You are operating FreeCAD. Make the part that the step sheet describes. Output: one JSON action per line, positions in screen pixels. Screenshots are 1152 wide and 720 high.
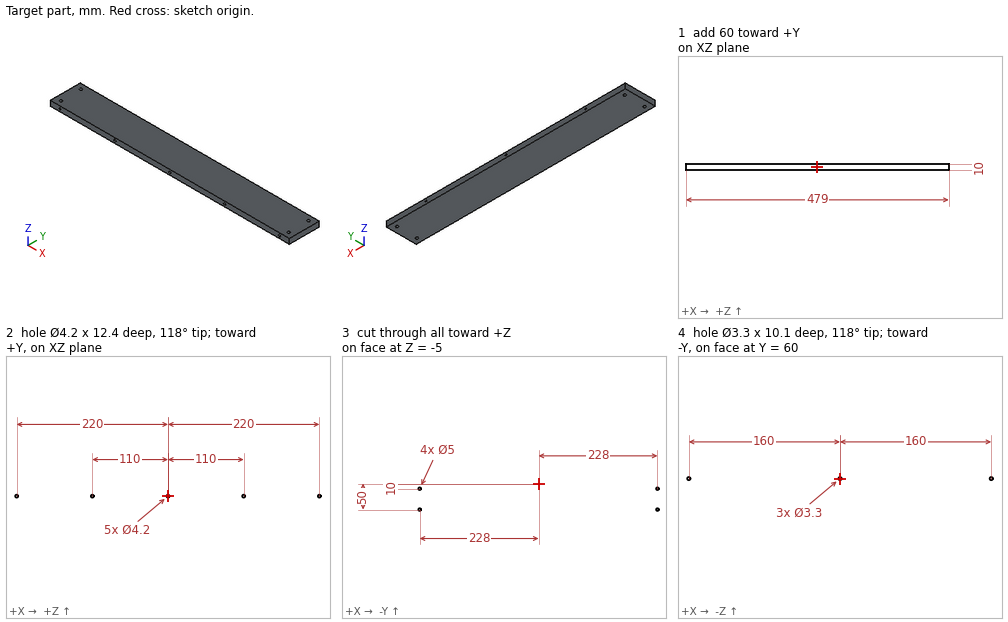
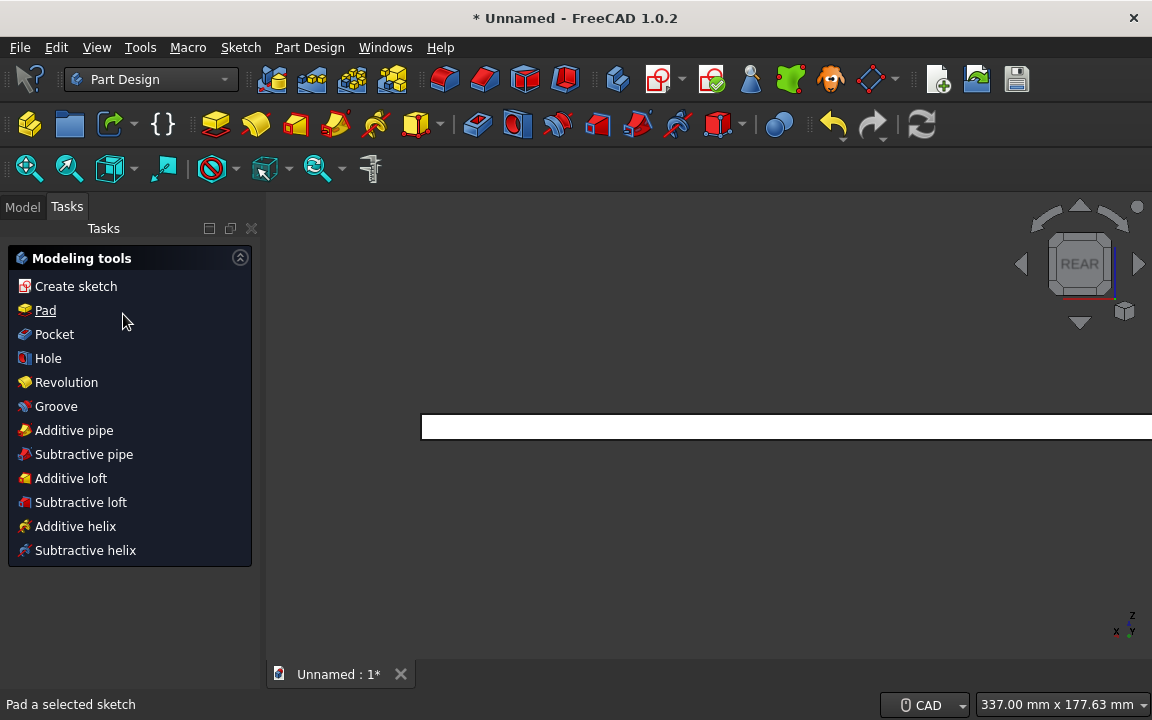
{"action": "left_click", "coordinate": [518, 124]}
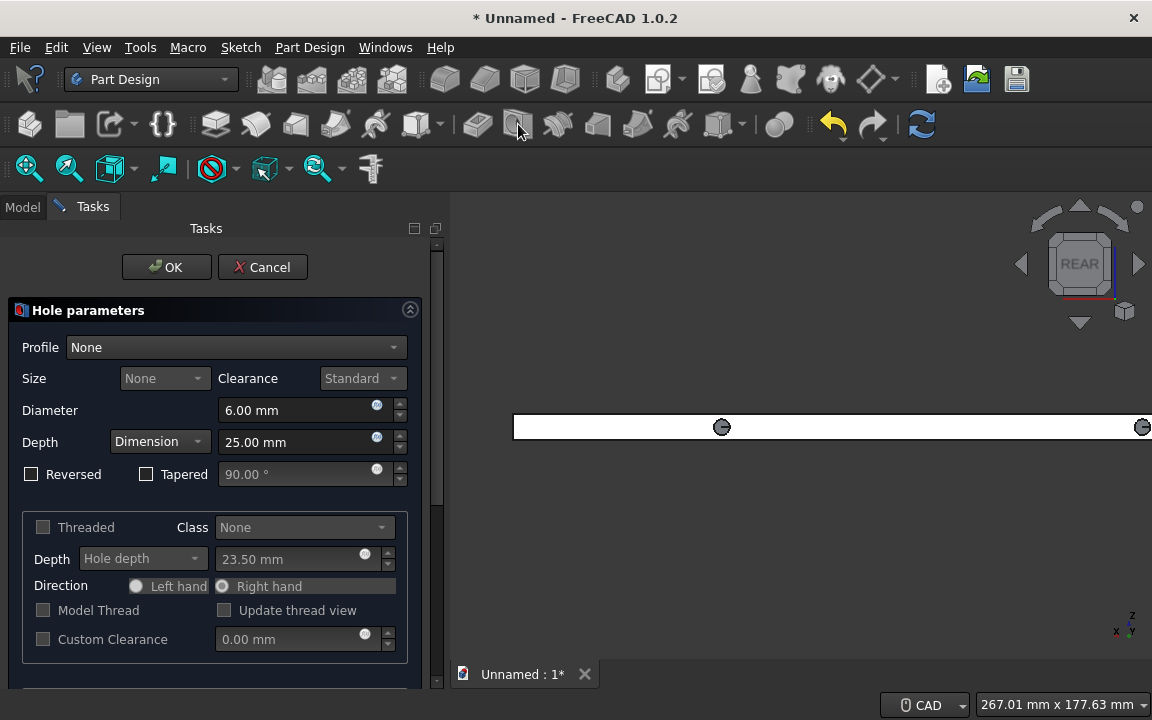
{"action": "triple_click", "coordinate": [305, 410]}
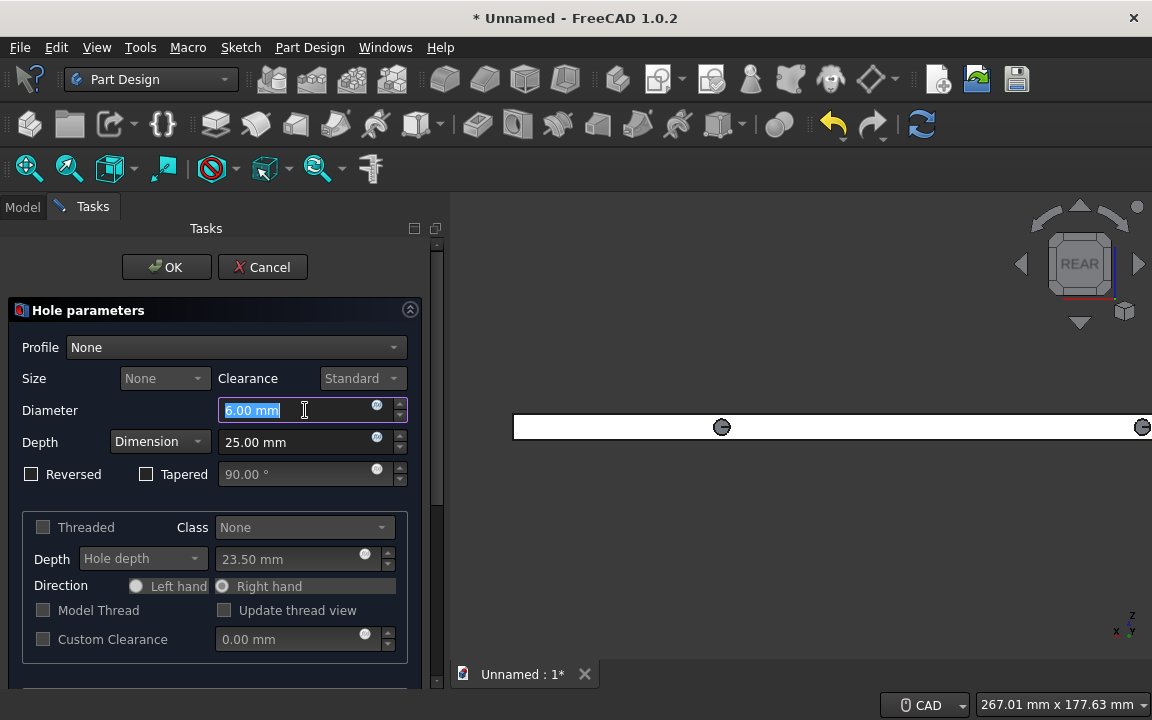
{"action": "type", "text": "3.3"}
{"action": "key", "text": "Tab"}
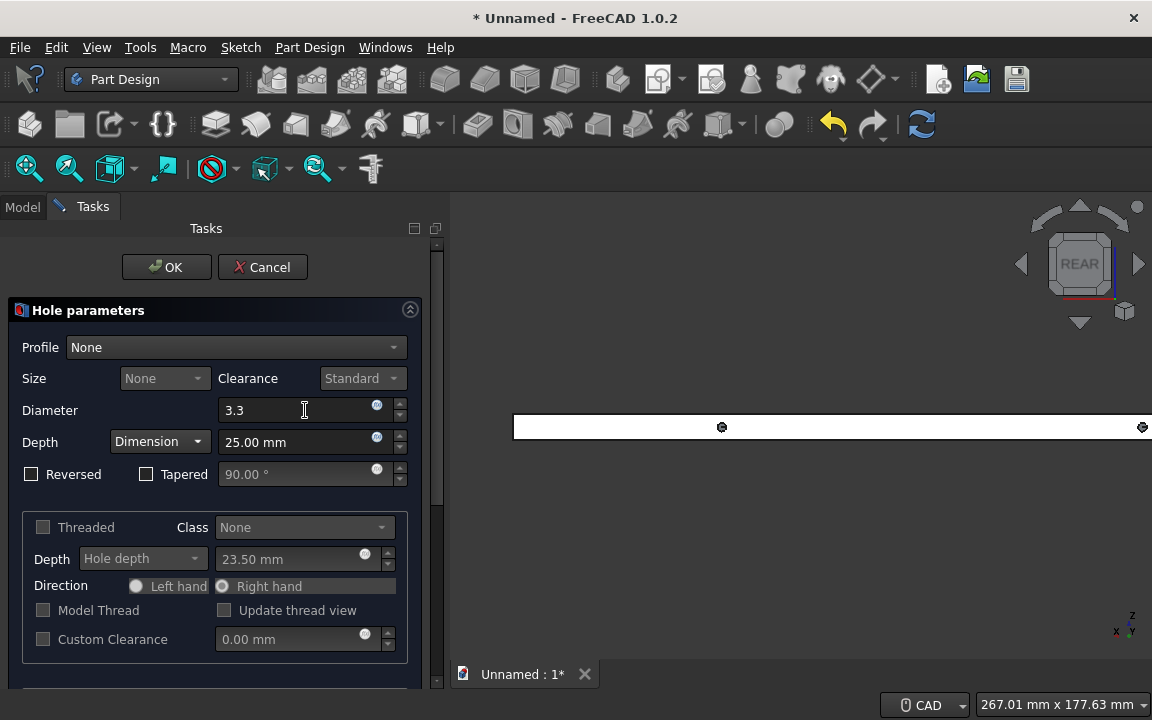
{"action": "triple_click", "coordinate": [305, 442]}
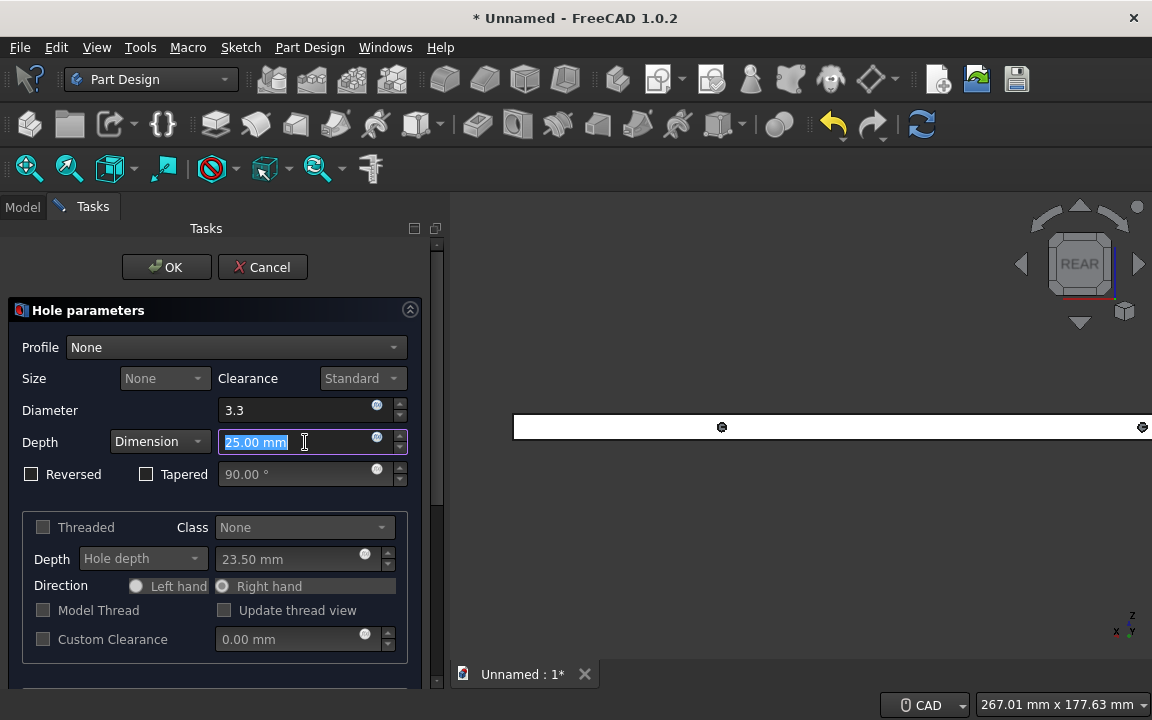
{"action": "type", "text": "10.1"}
{"action": "key", "text": "Tab"}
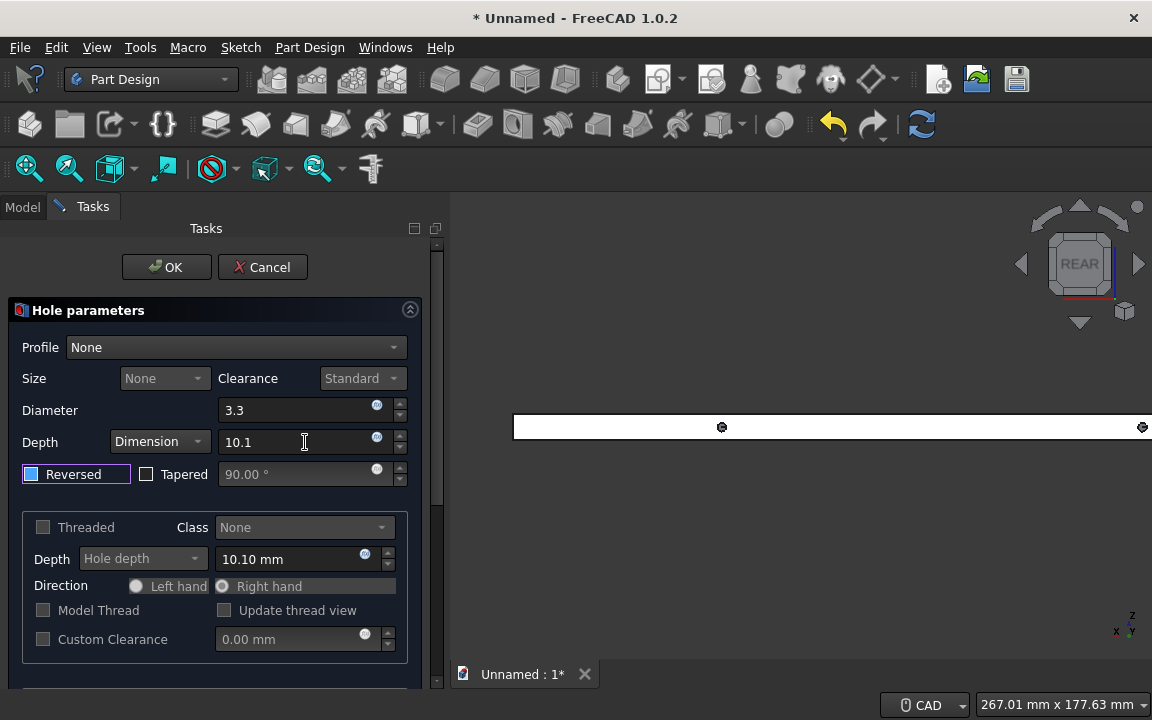
{"action": "left_click", "coordinate": [167, 267]}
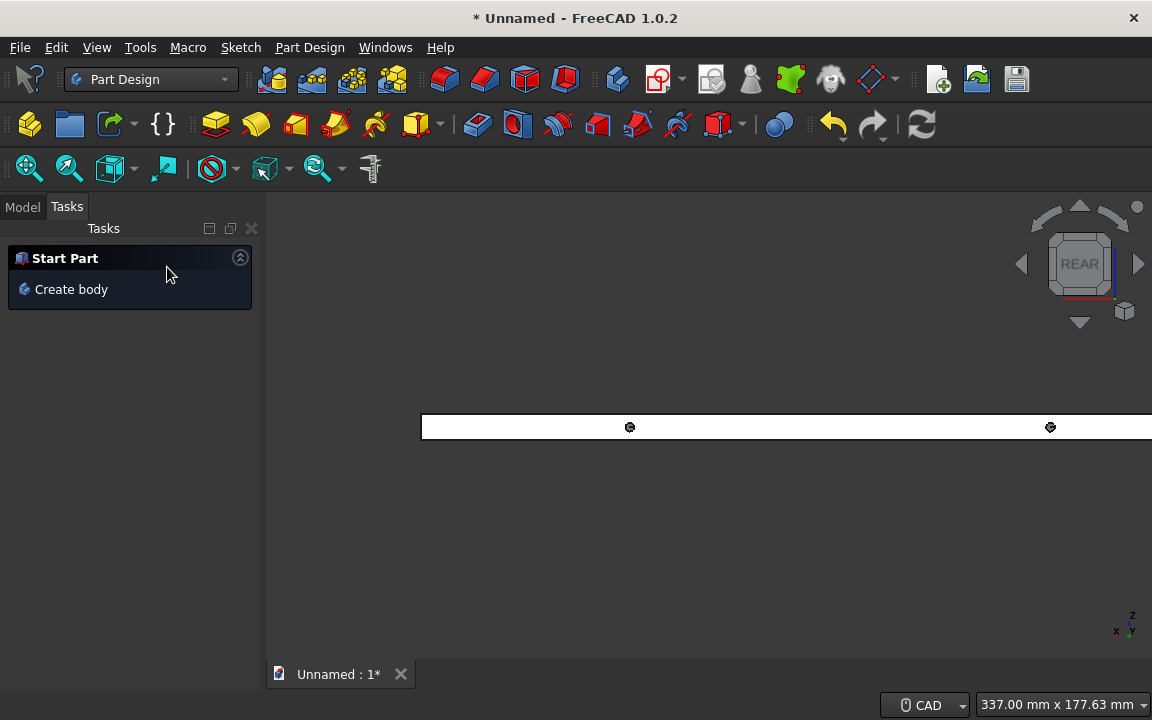
{"action": "key", "text": "0"}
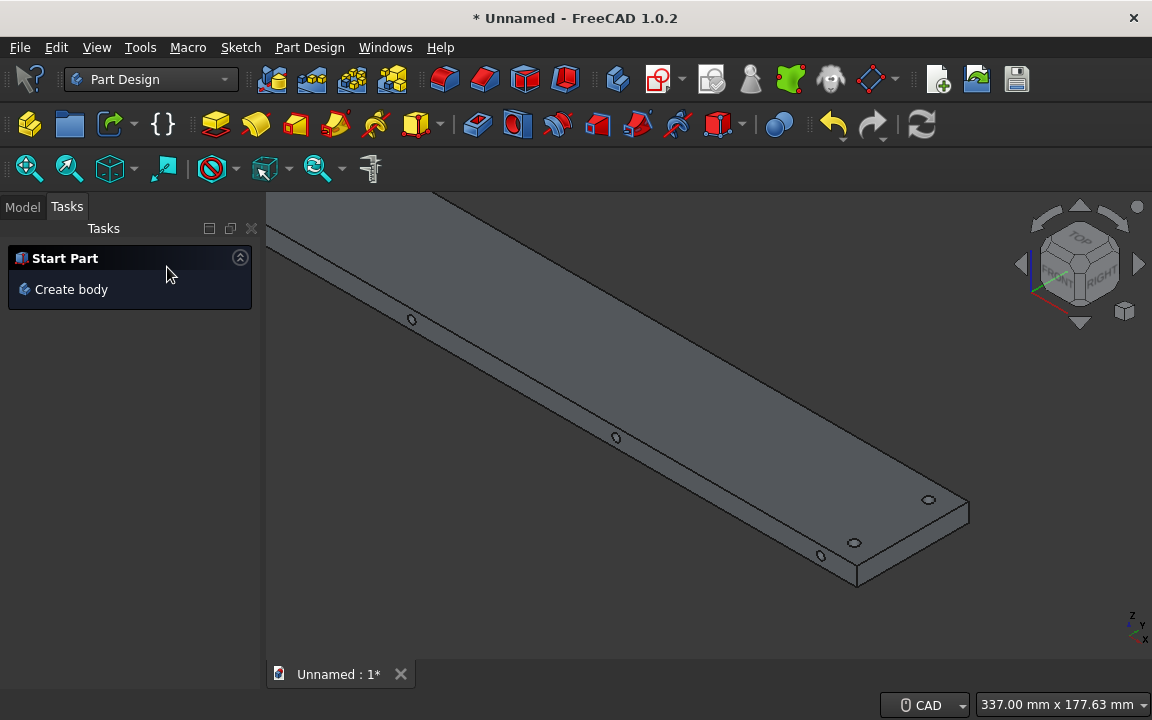
{"action": "key", "text": "v f"}